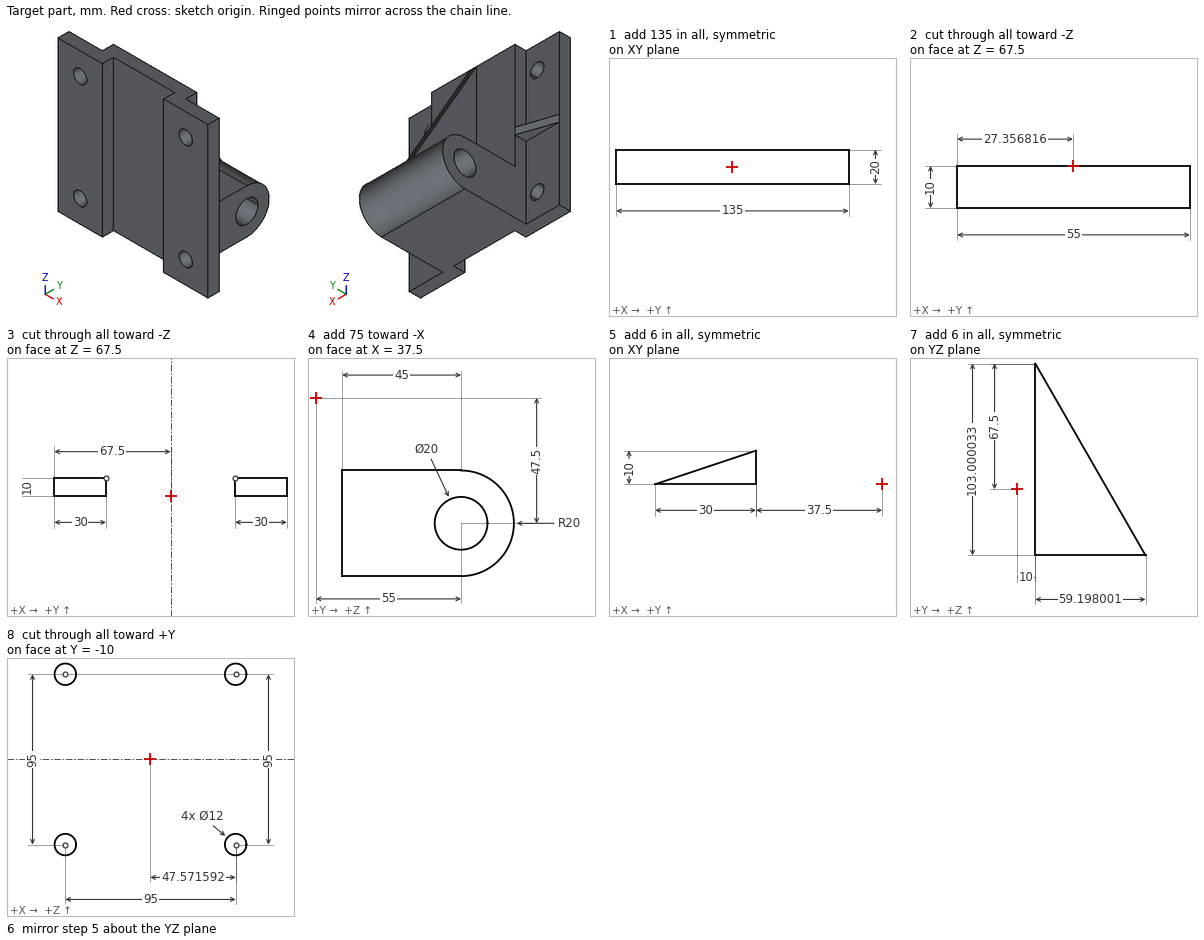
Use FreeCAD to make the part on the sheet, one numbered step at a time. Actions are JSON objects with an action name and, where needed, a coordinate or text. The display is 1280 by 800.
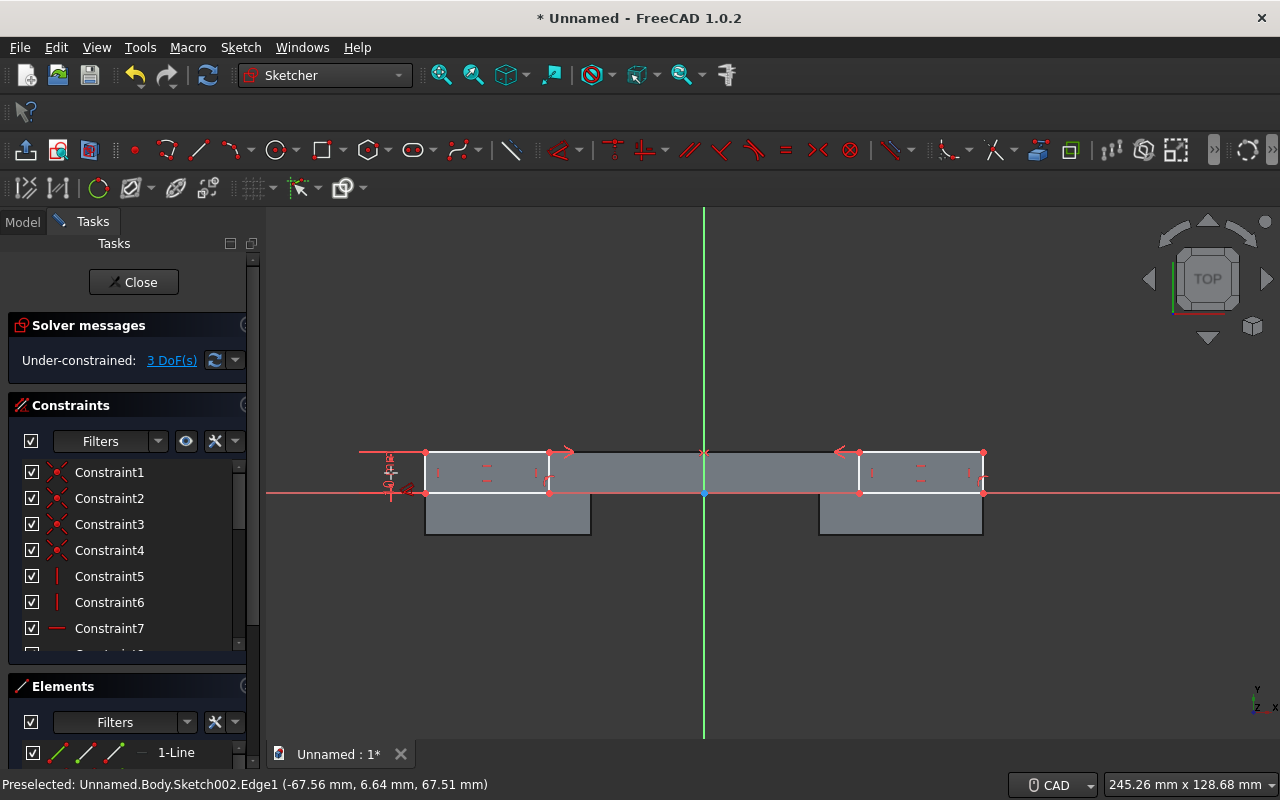
{"action": "left_click", "coordinate": [462, 493]}
{"action": "left_click", "coordinate": [487, 527]}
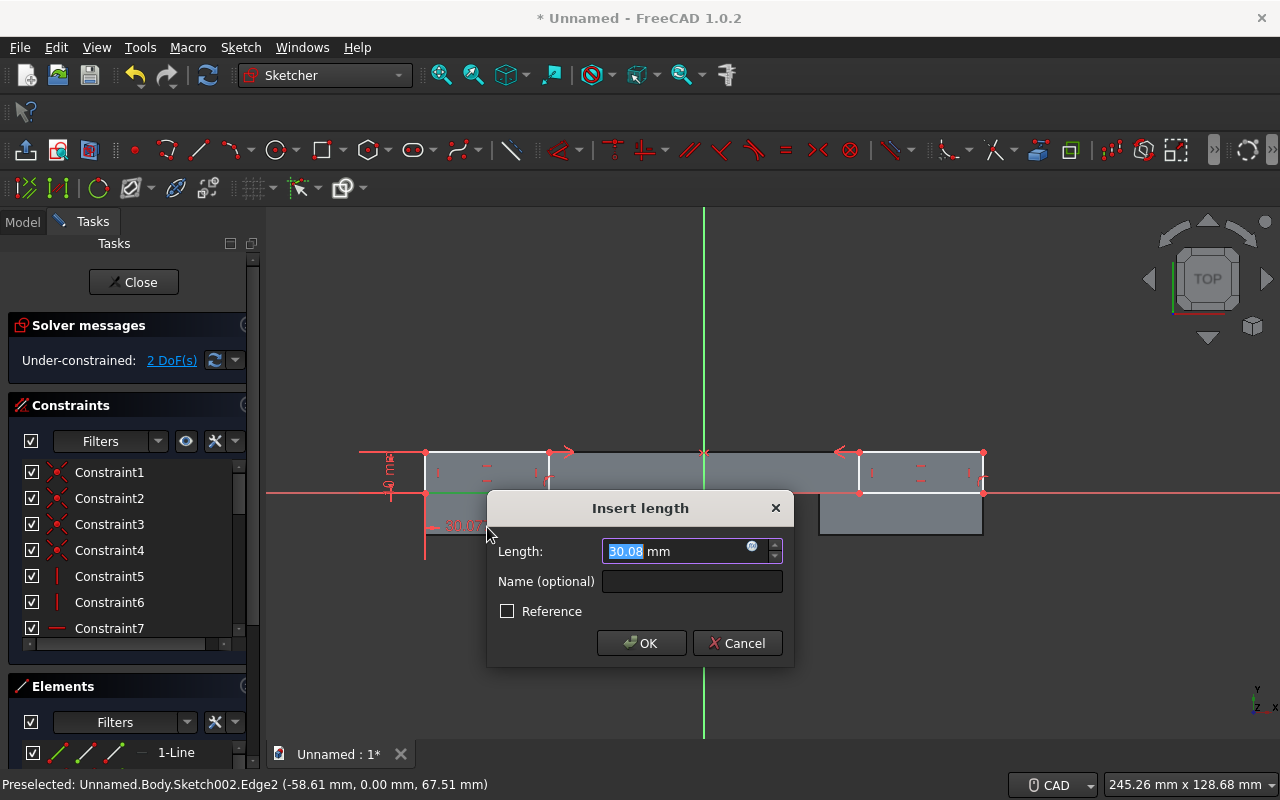
{"action": "type", "text": "30"}
{"action": "key", "text": "Return"}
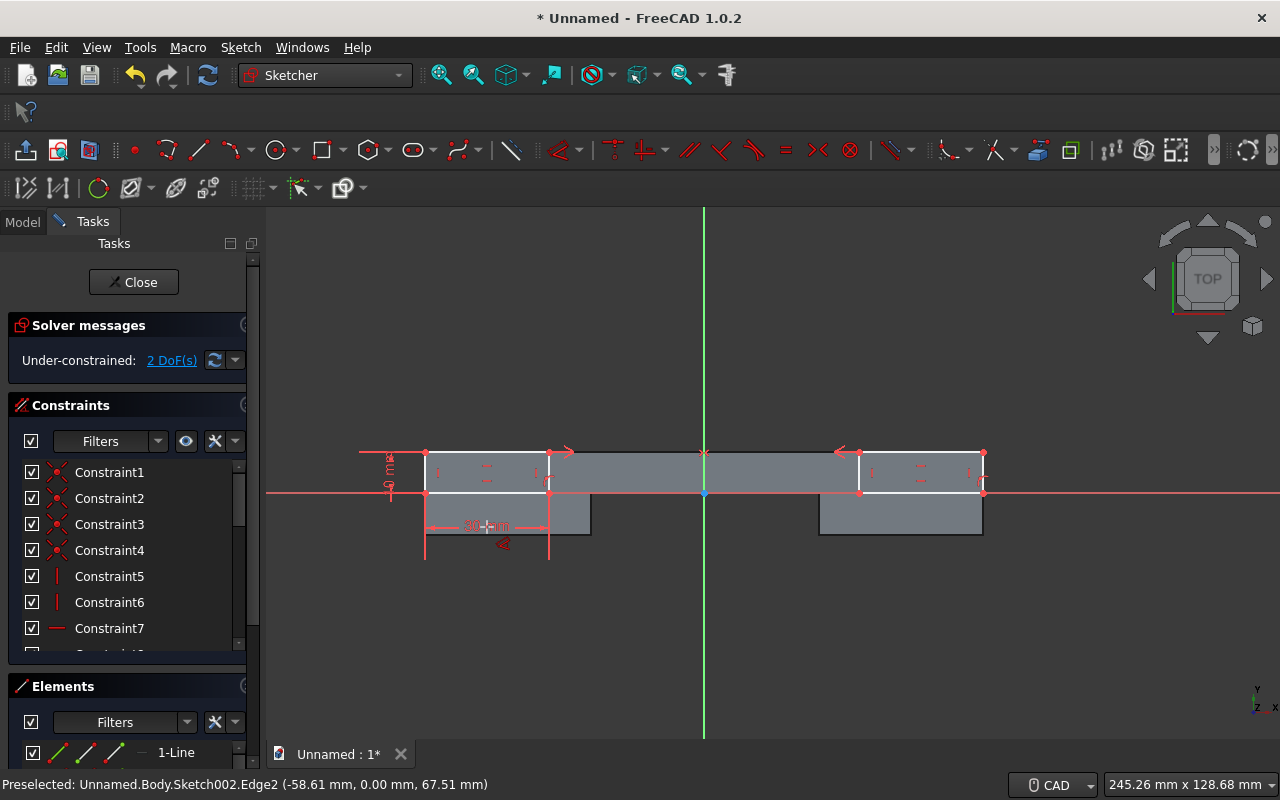
{"action": "left_click", "coordinate": [896, 493]}
{"action": "left_click", "coordinate": [921, 527]}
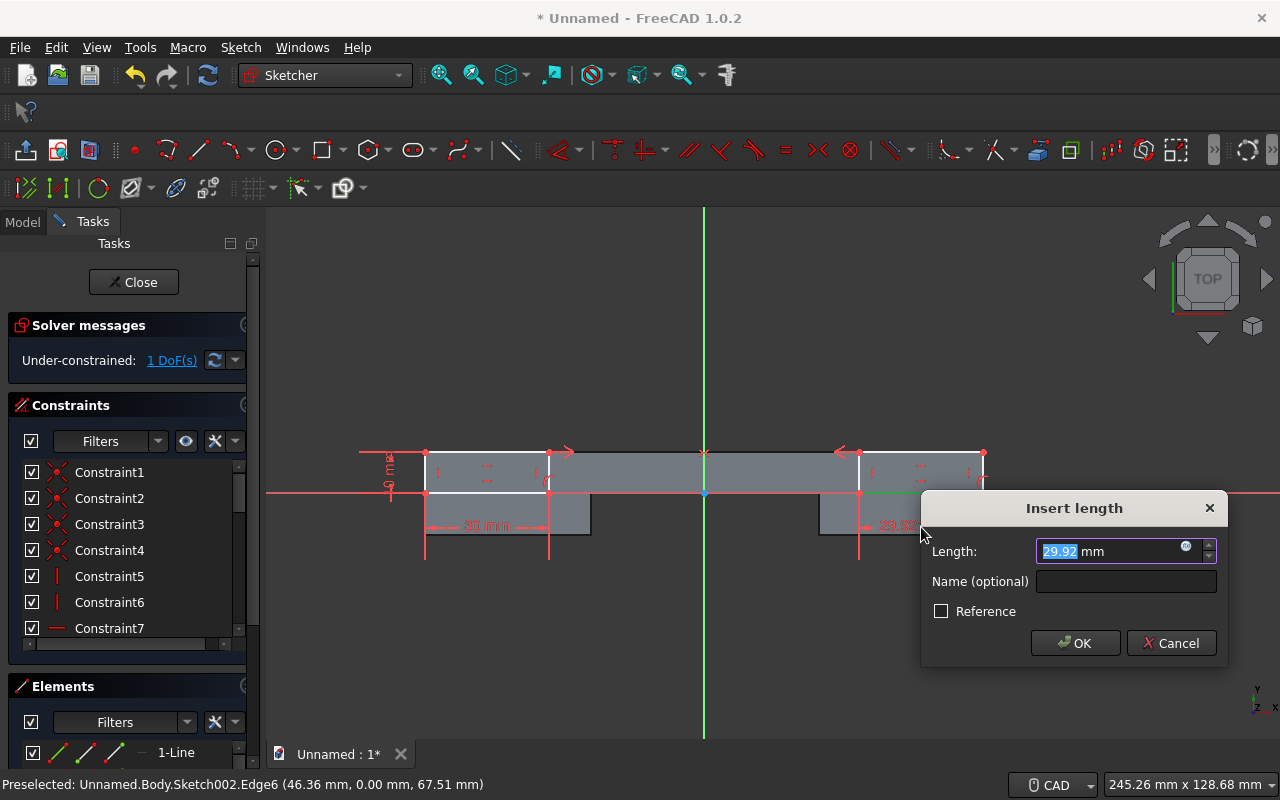
{"action": "type", "text": "30"}
{"action": "key", "text": "Return"}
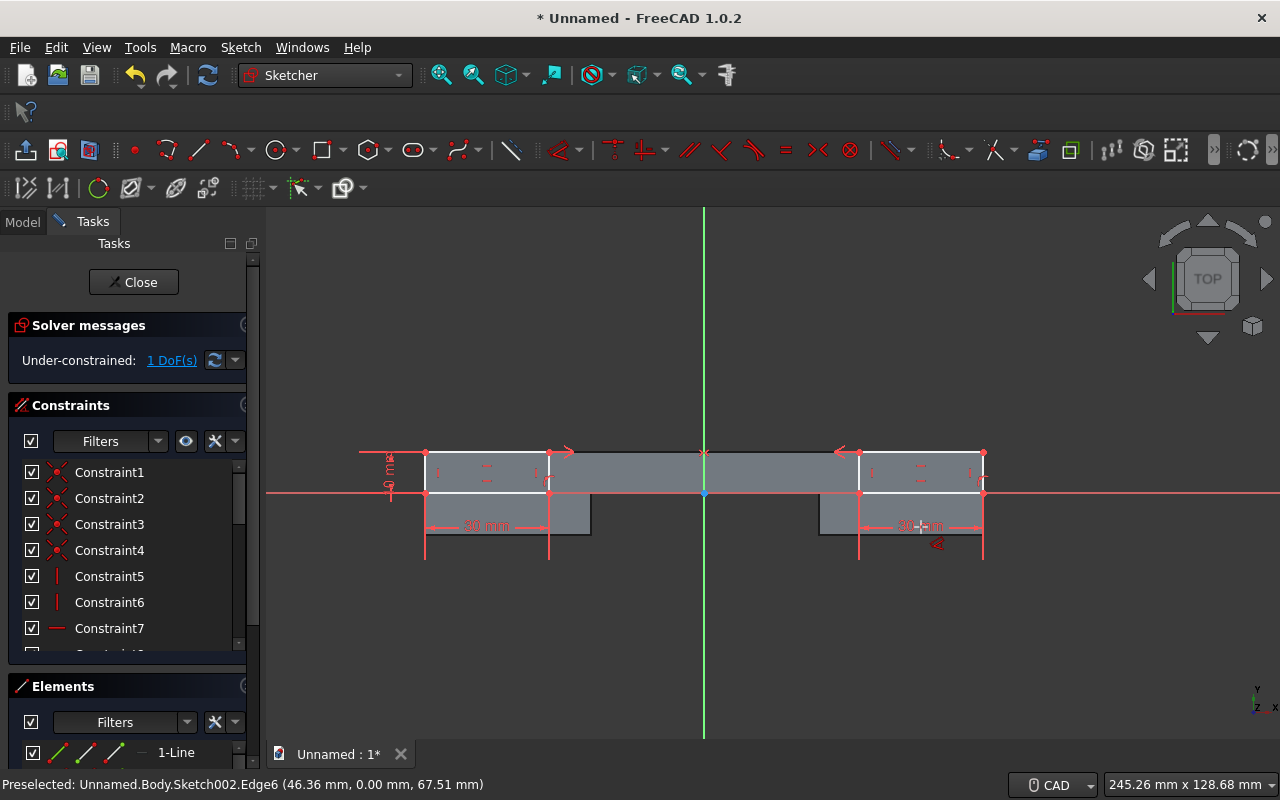
{"action": "left_click", "coordinate": [425, 452]}
{"action": "left_click", "coordinate": [565, 527]}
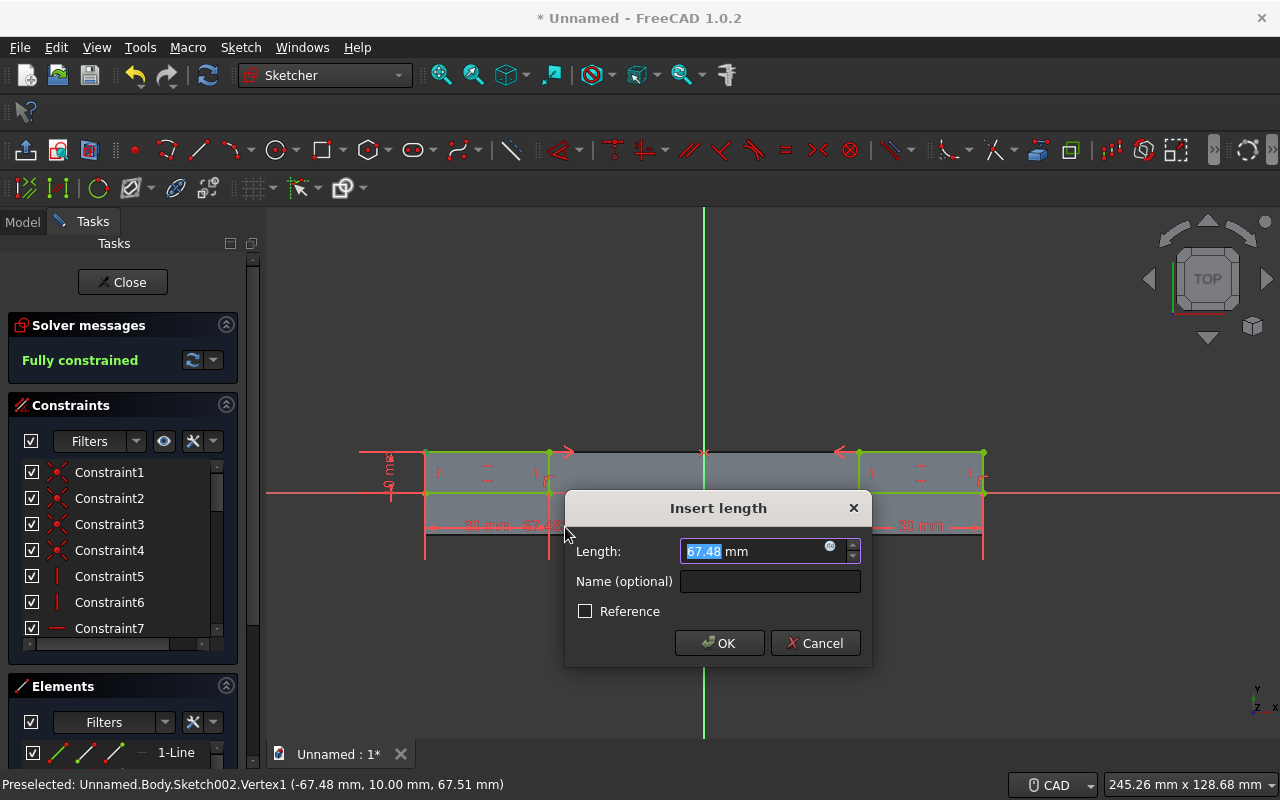
{"action": "type", "text": "67.5"}
{"action": "key", "text": "Return"}
{"action": "key", "text": "Escape"}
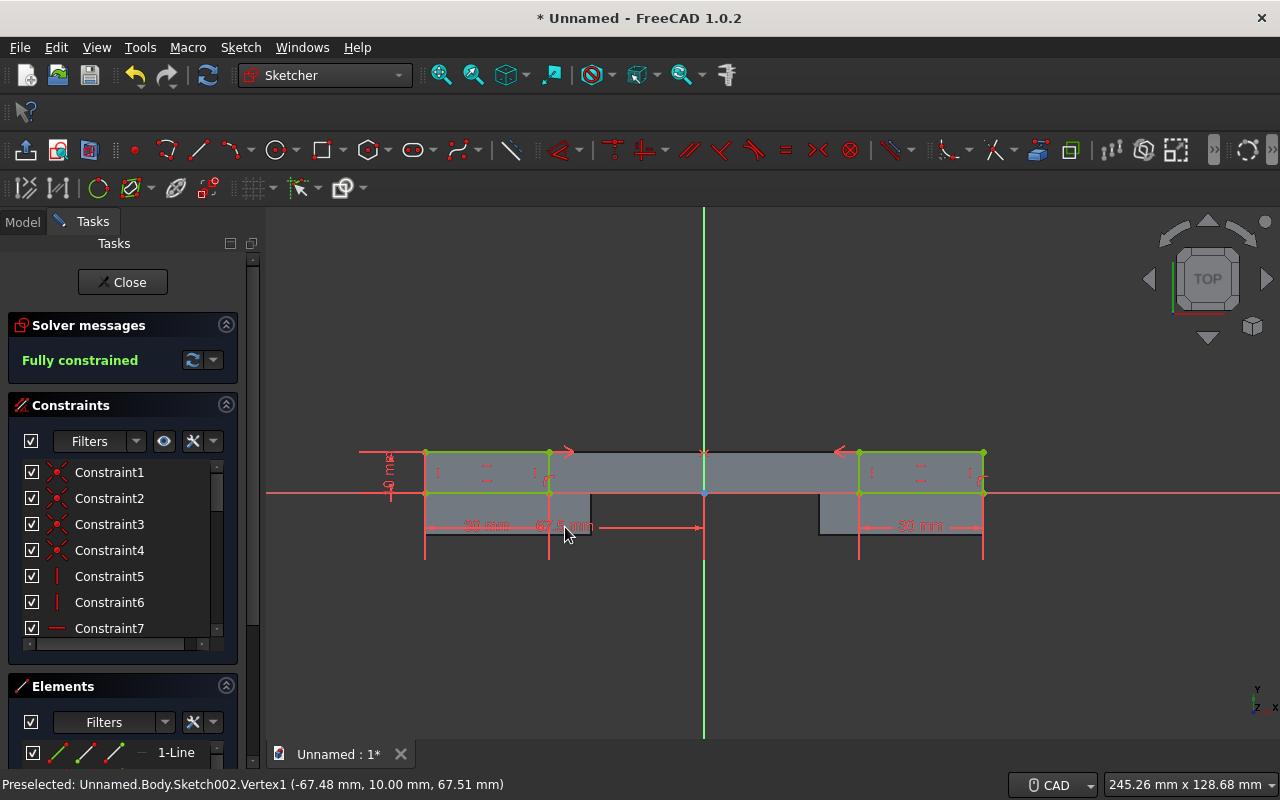
{"action": "left_click", "coordinate": [123, 282]}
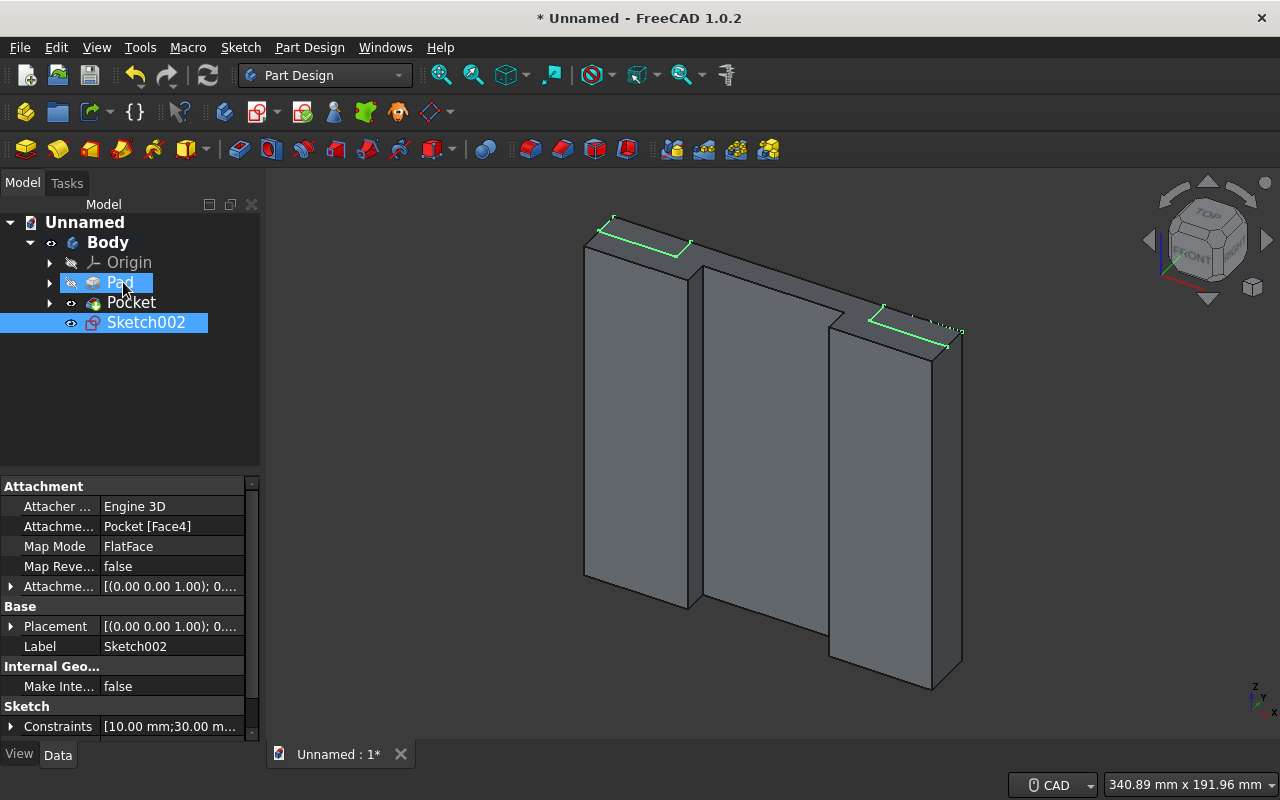
{"action": "left_click", "coordinate": [240, 150]}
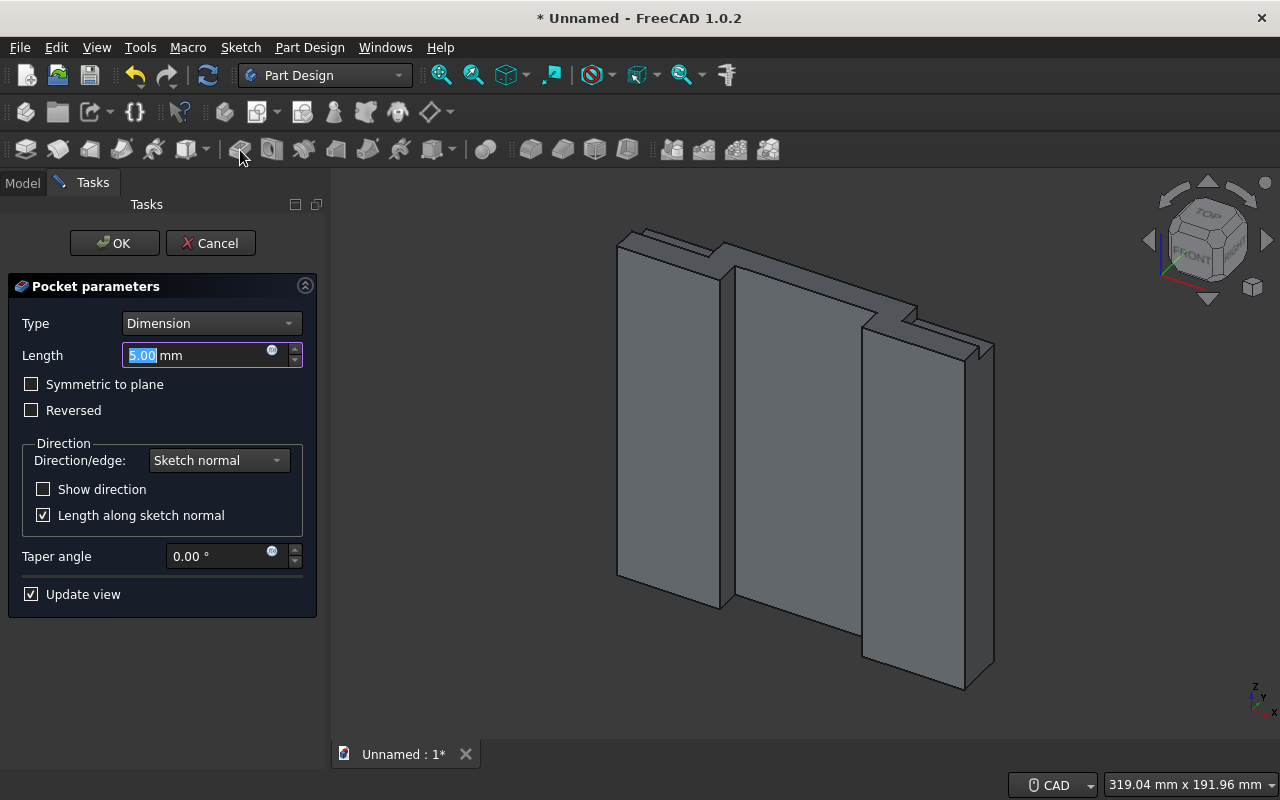
{"action": "left_click", "coordinate": [212, 324]}